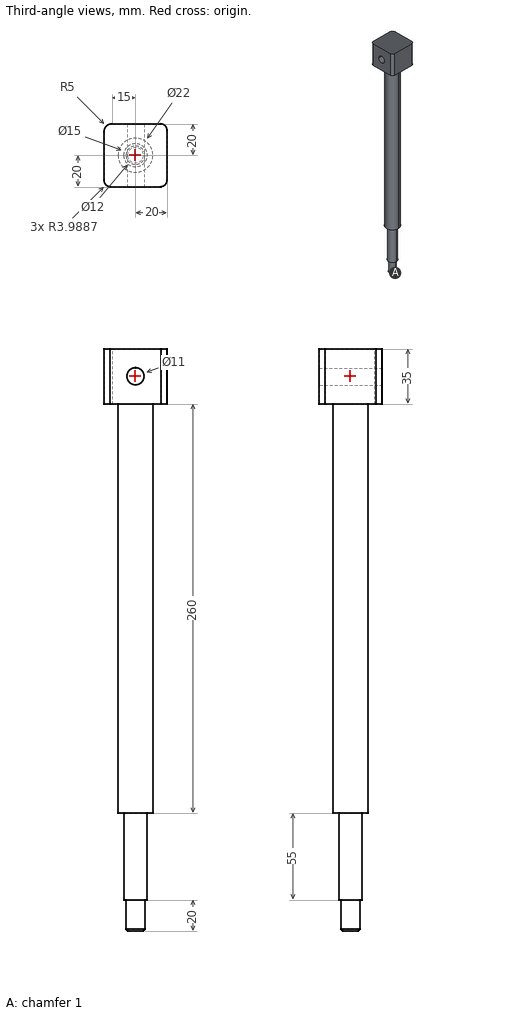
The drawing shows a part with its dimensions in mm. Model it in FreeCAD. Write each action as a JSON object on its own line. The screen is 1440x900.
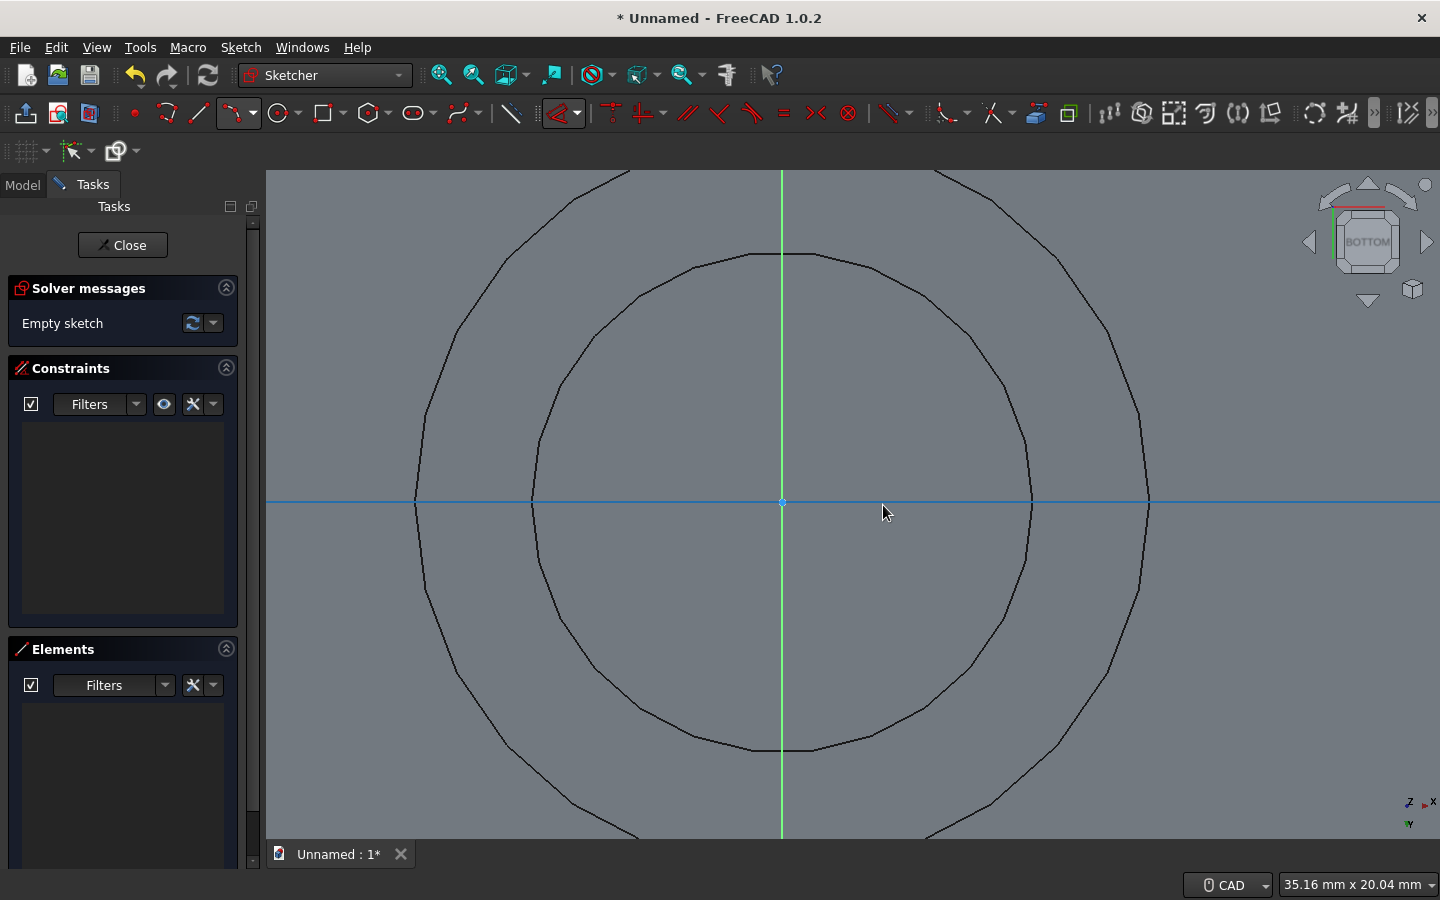
{"action": "left_click", "coordinate": [278, 114]}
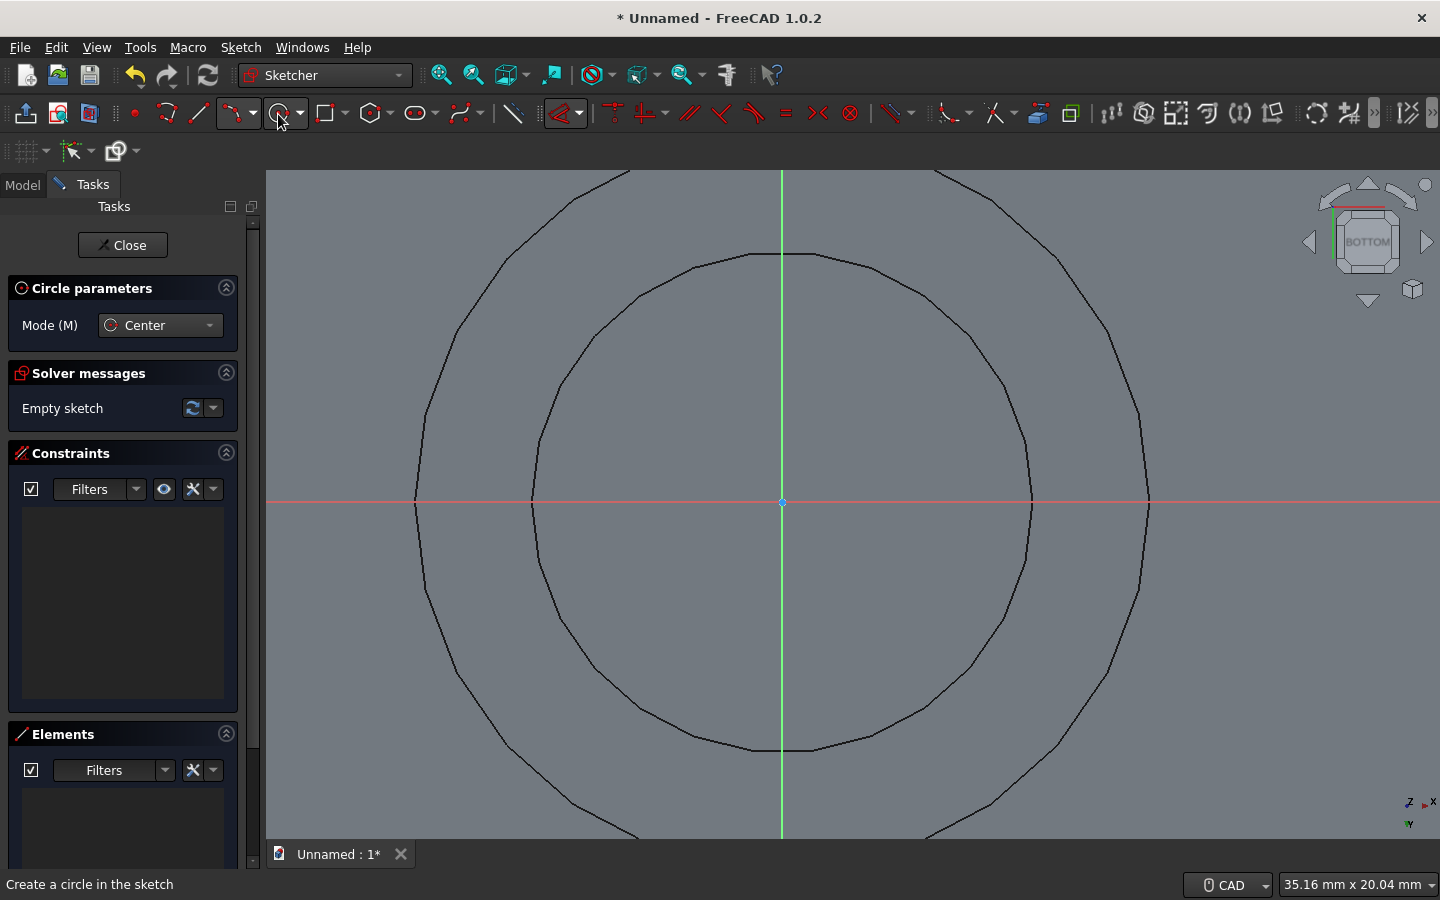
{"action": "left_click", "coordinate": [782, 502]}
{"action": "left_click", "coordinate": [924, 361]}
{"action": "key", "text": "Escape"}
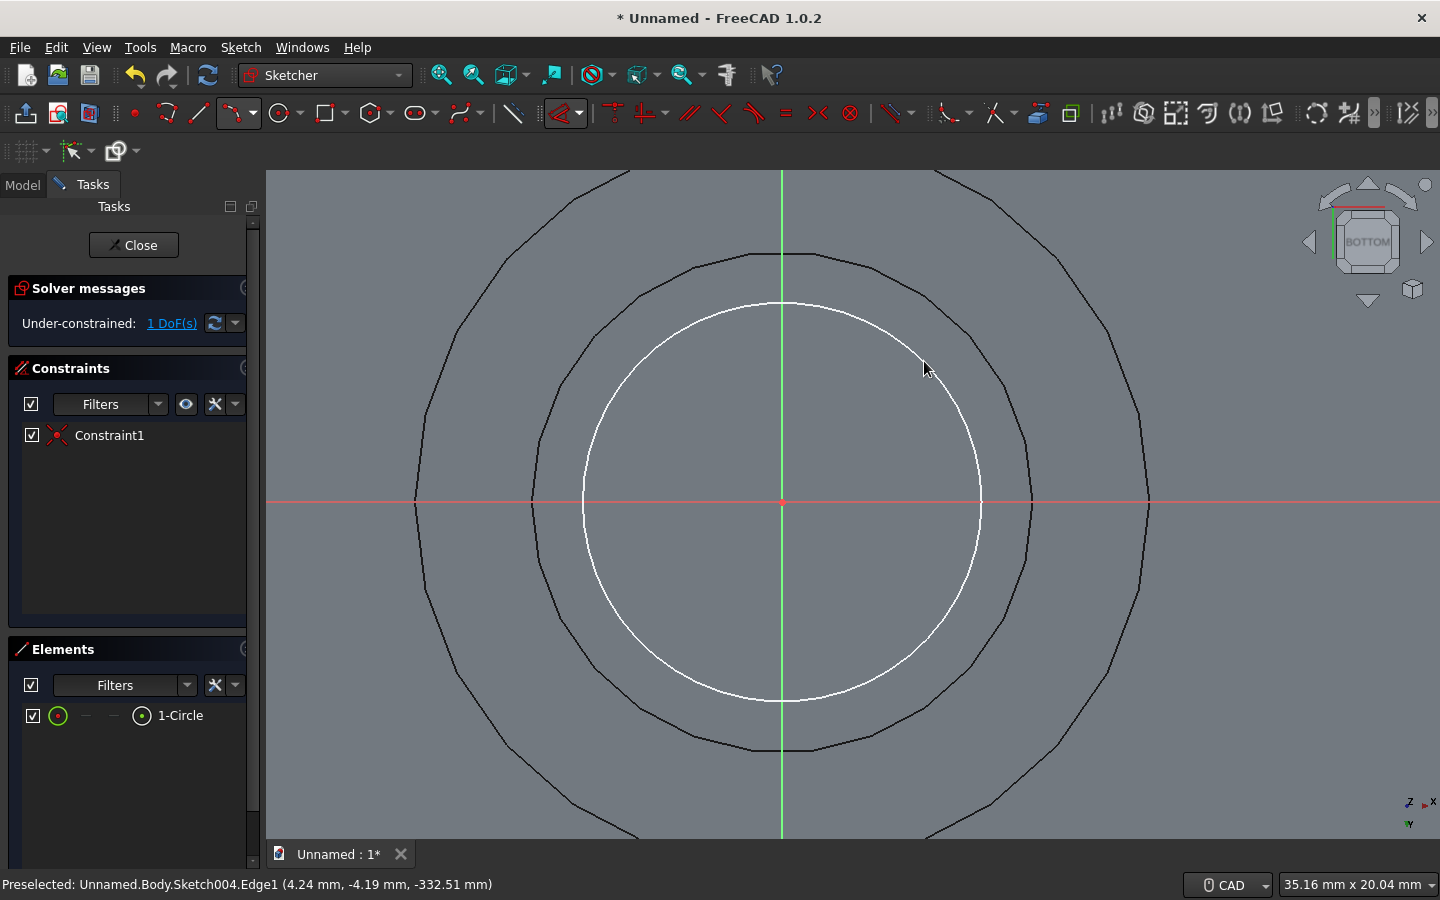
{"action": "left_click", "coordinate": [923, 361]}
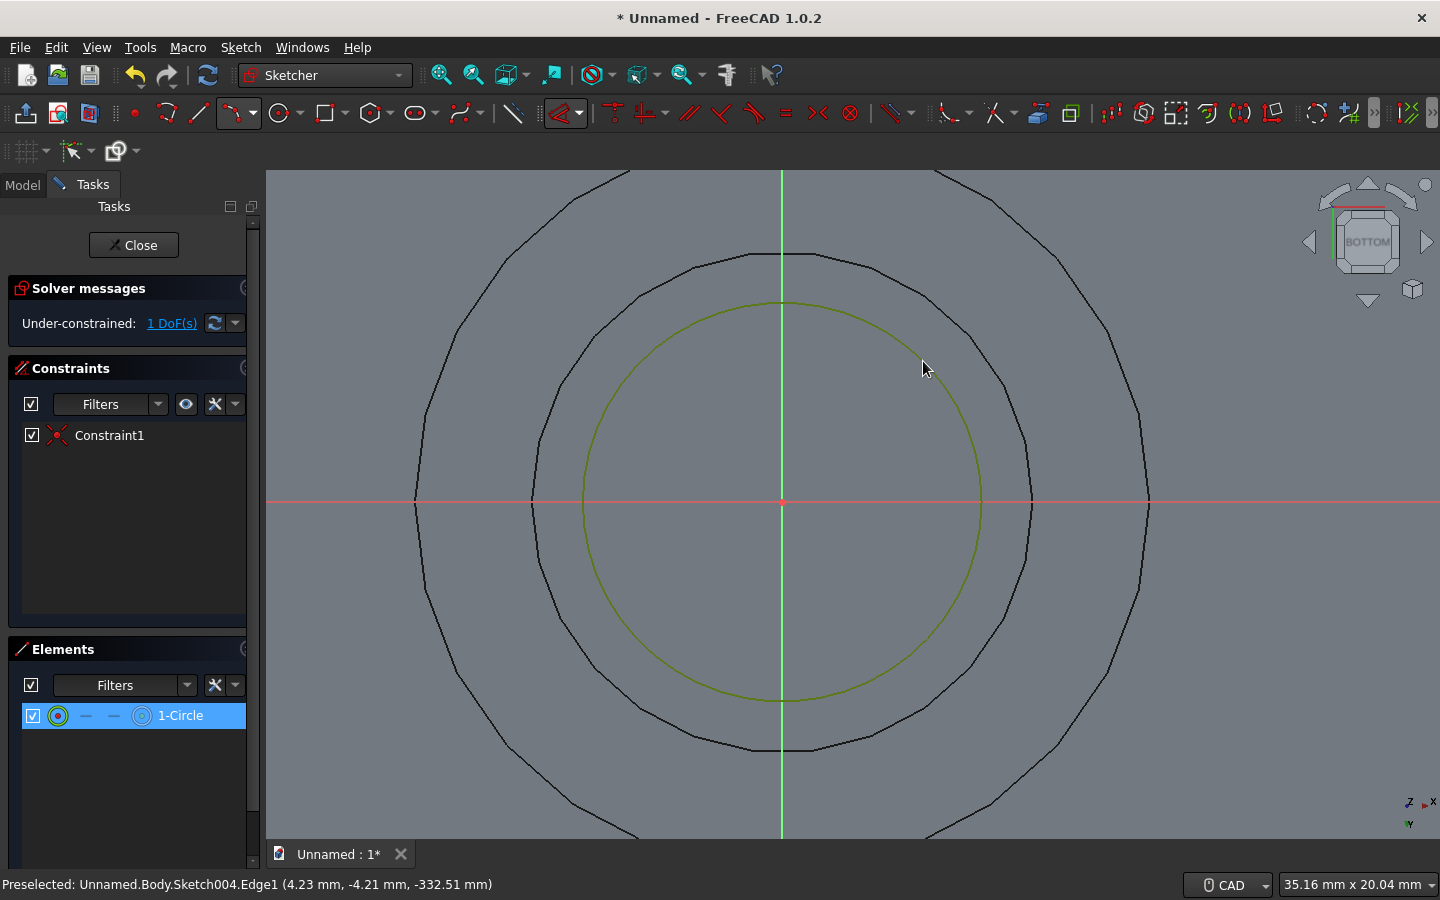
{"action": "key", "text": "k o"}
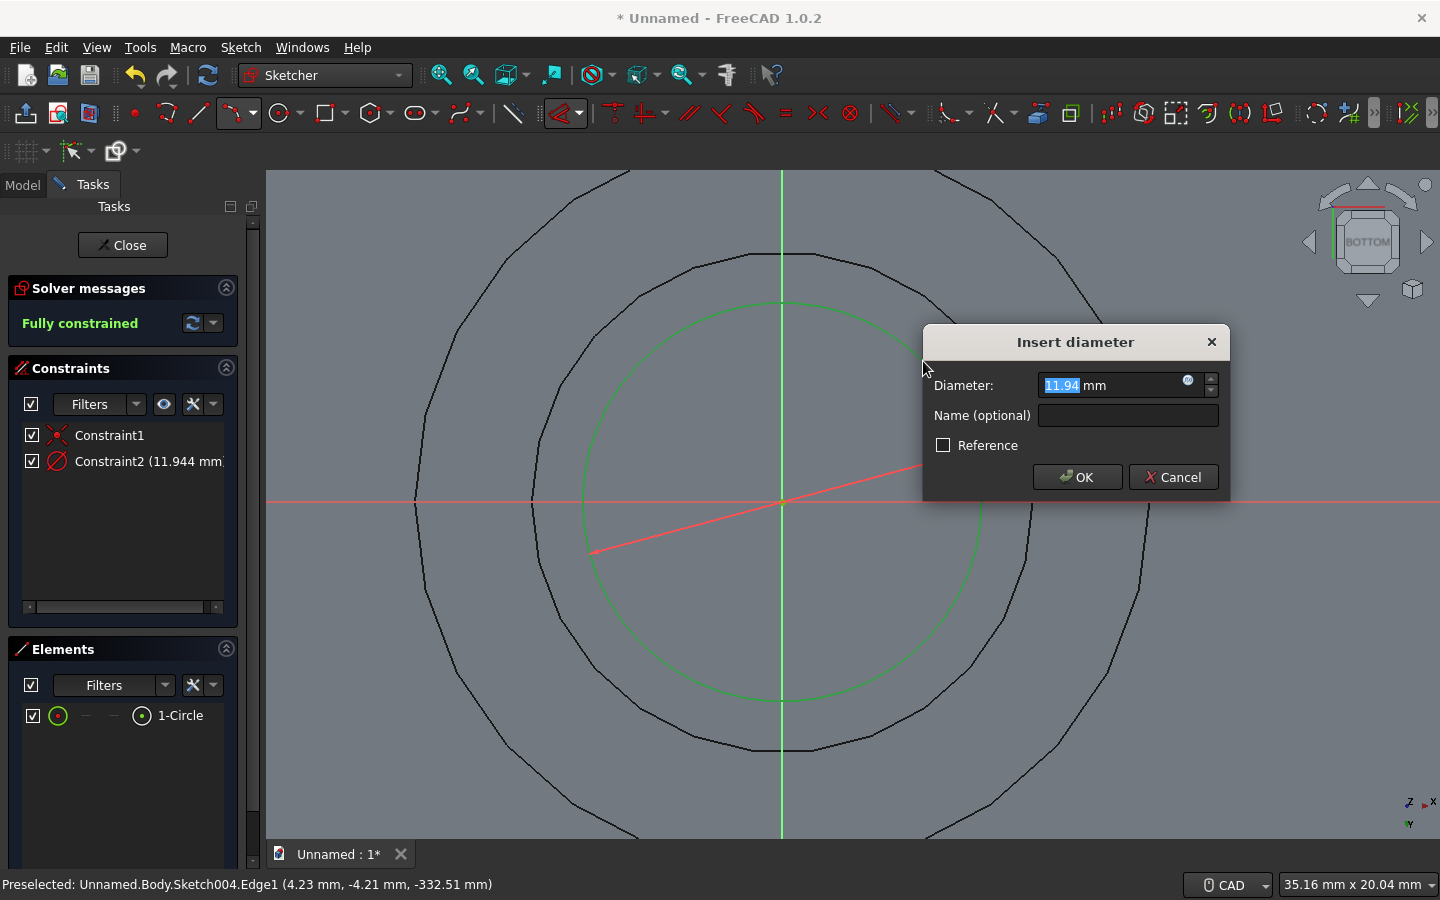
{"action": "type", "text": "12"}
{"action": "key", "text": "Return"}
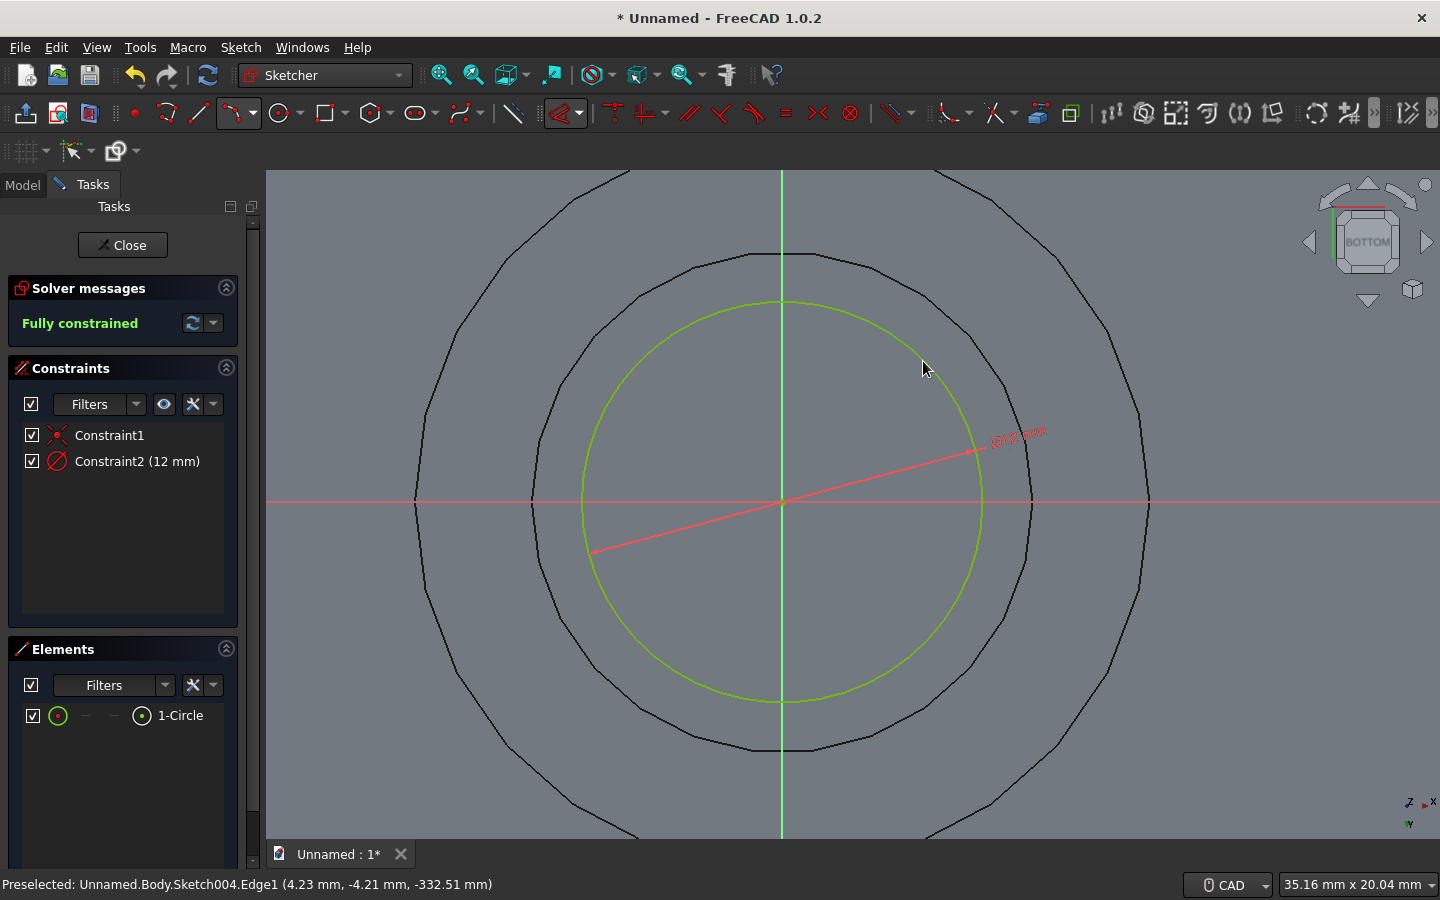
{"action": "left_click", "coordinate": [123, 245]}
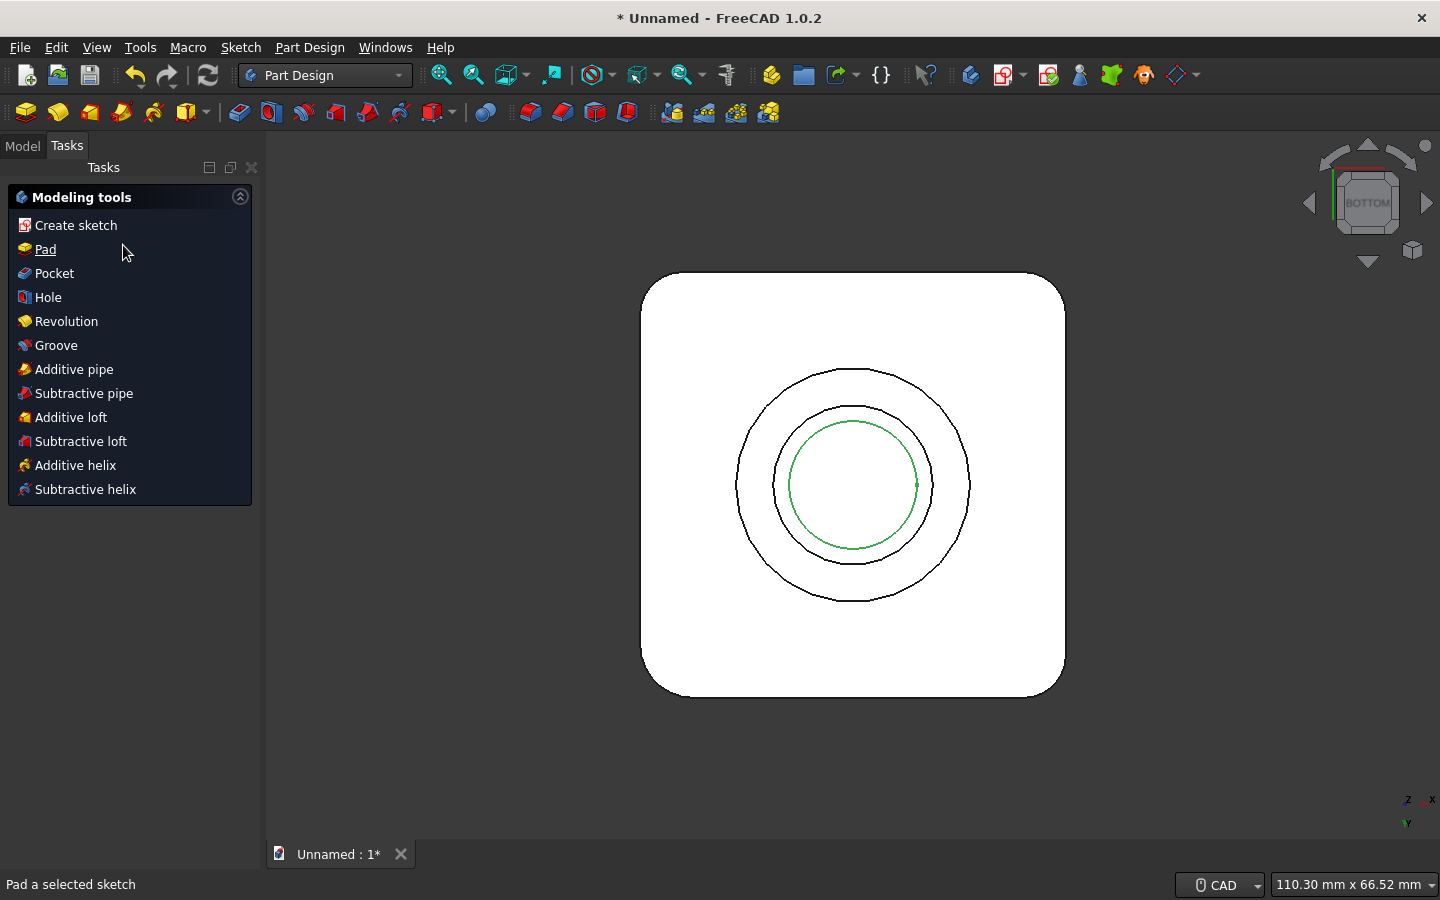
{"action": "left_click", "coordinate": [26, 112]}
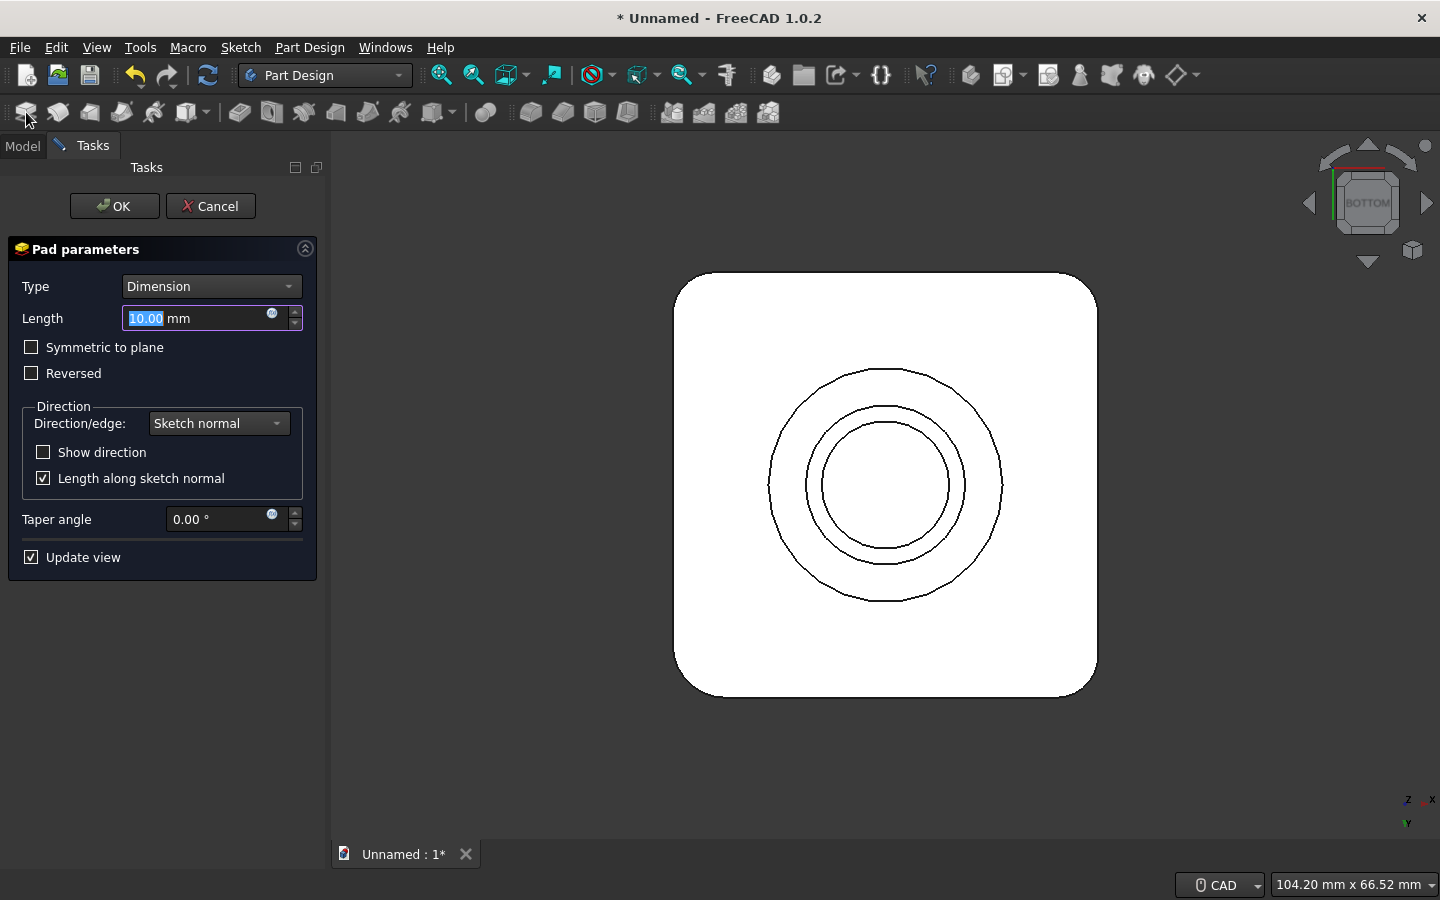
{"action": "type", "text": "20"}
{"action": "key", "text": "Tab"}